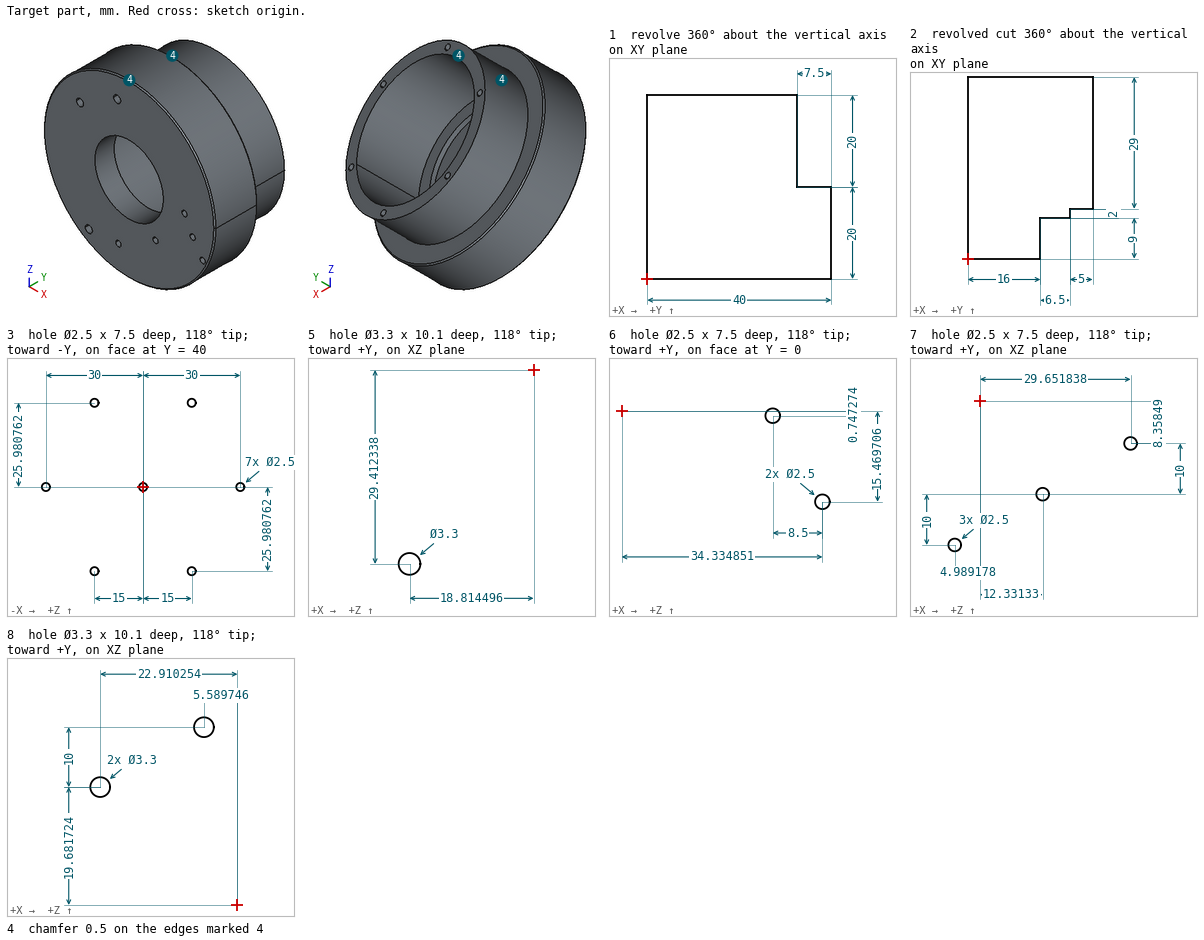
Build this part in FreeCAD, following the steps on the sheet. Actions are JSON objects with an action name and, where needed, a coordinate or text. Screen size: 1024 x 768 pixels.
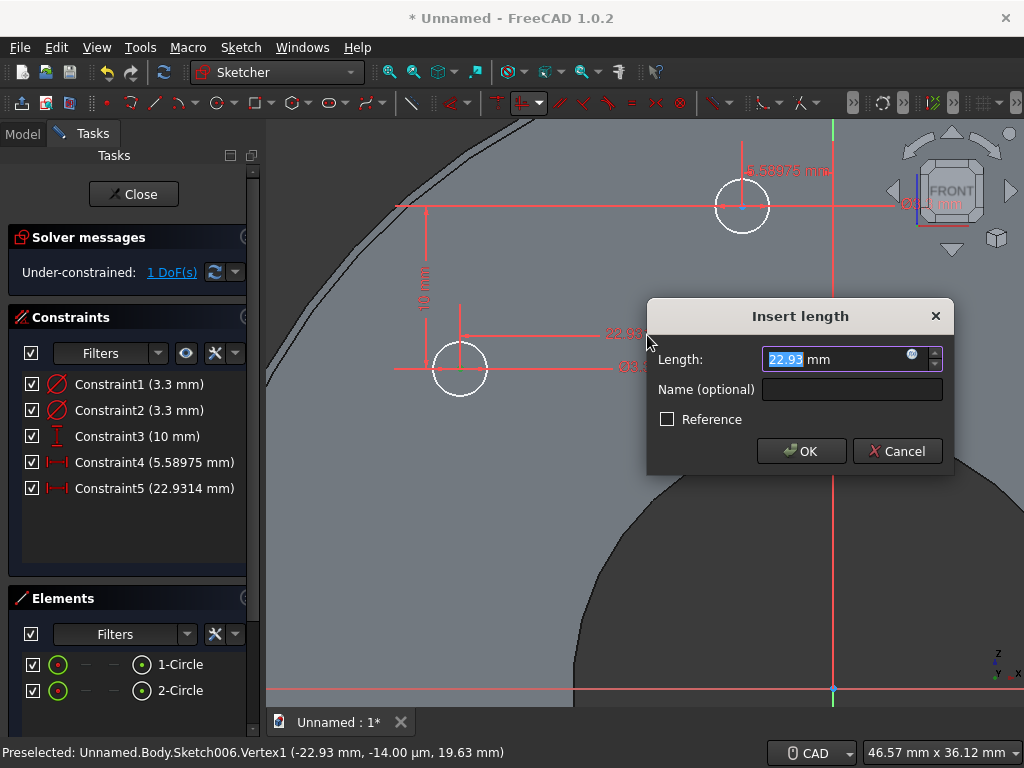
{"action": "type", "text": "22.910254"}
{"action": "key", "text": "Return"}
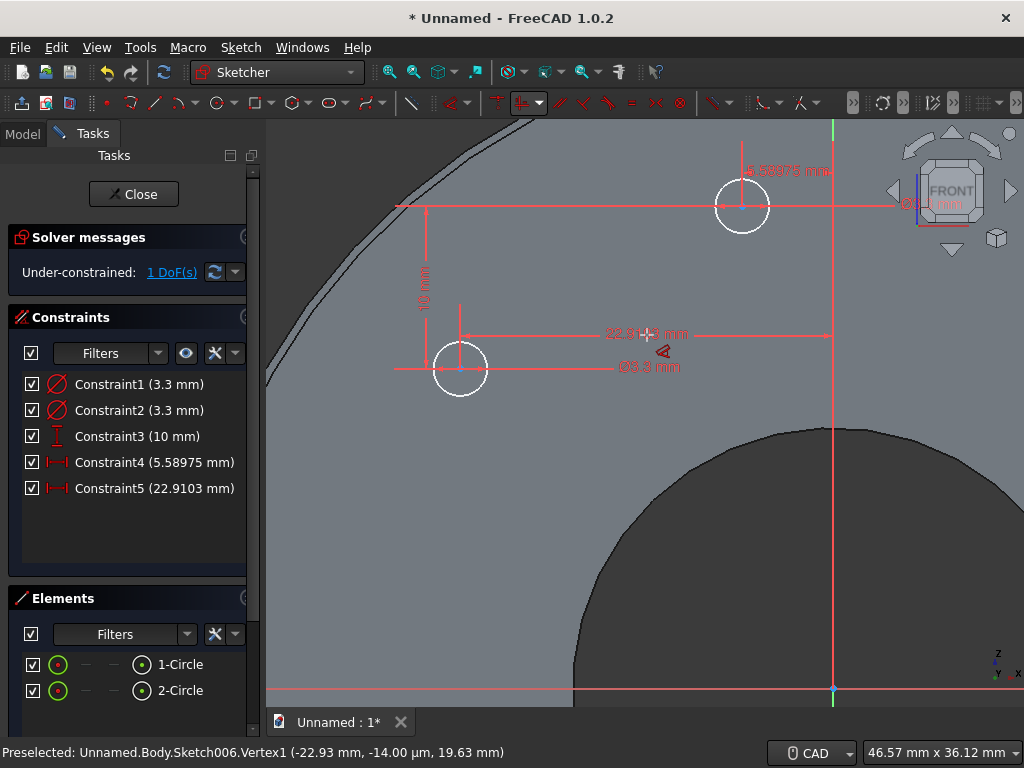
{"action": "left_click", "coordinate": [460, 369]}
{"action": "left_click", "coordinate": [426, 524]}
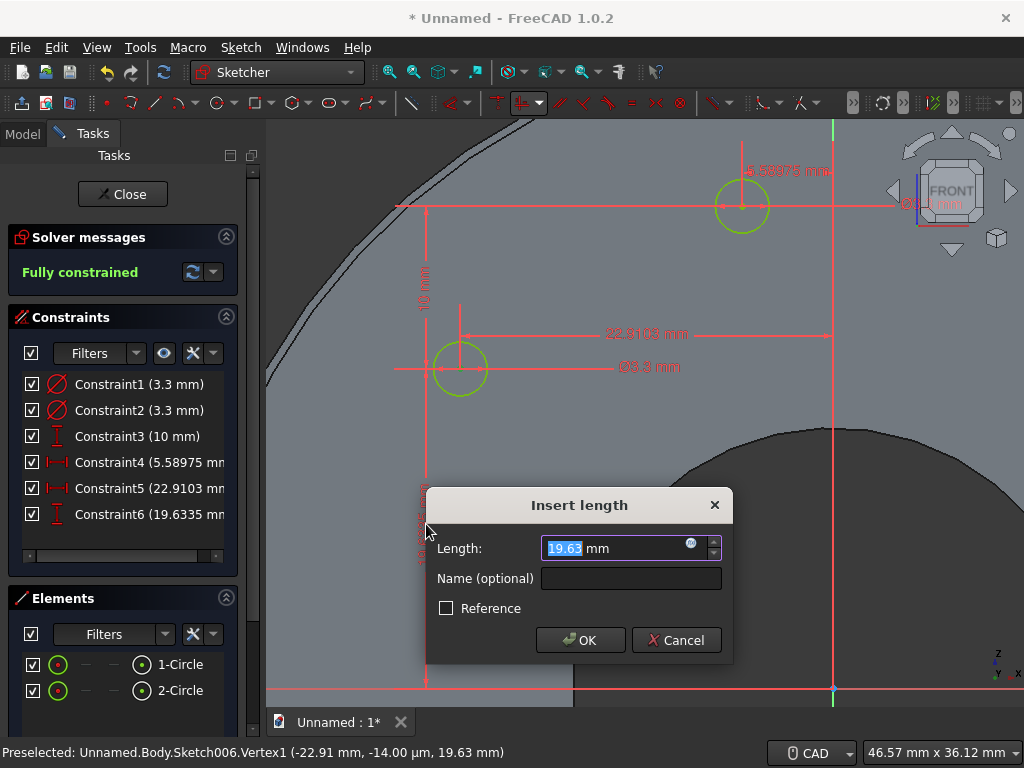
{"action": "type", "text": "19.681724"}
{"action": "key", "text": "Return"}
{"action": "key", "text": "Escape"}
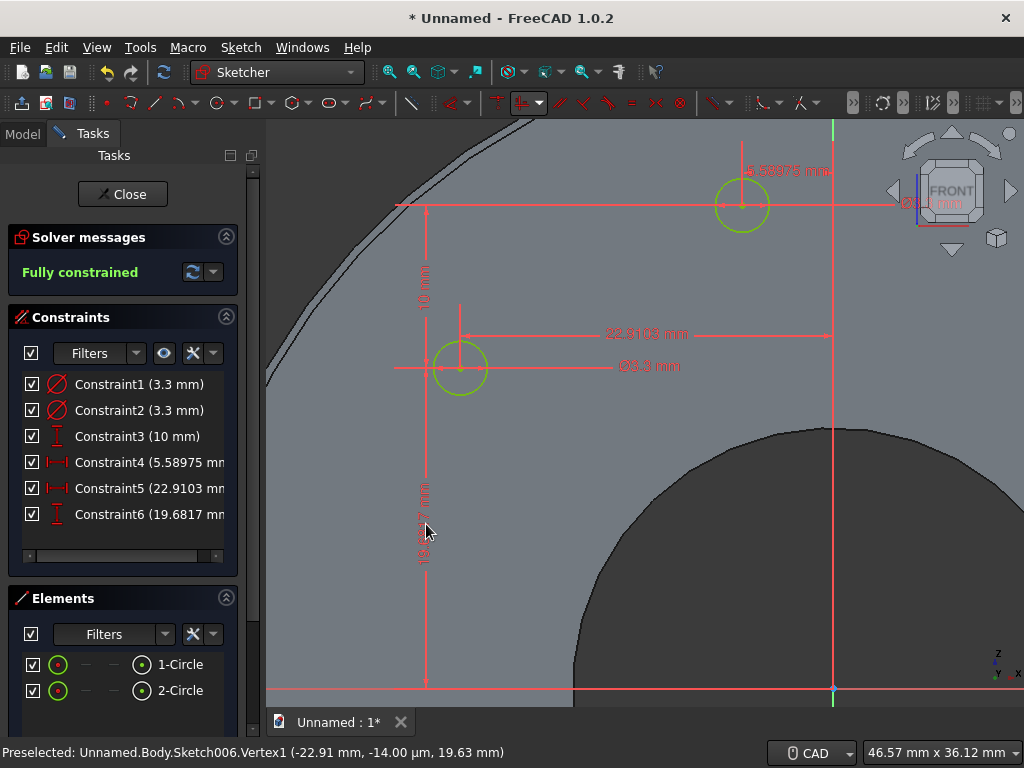
{"action": "left_click", "coordinate": [123, 194]}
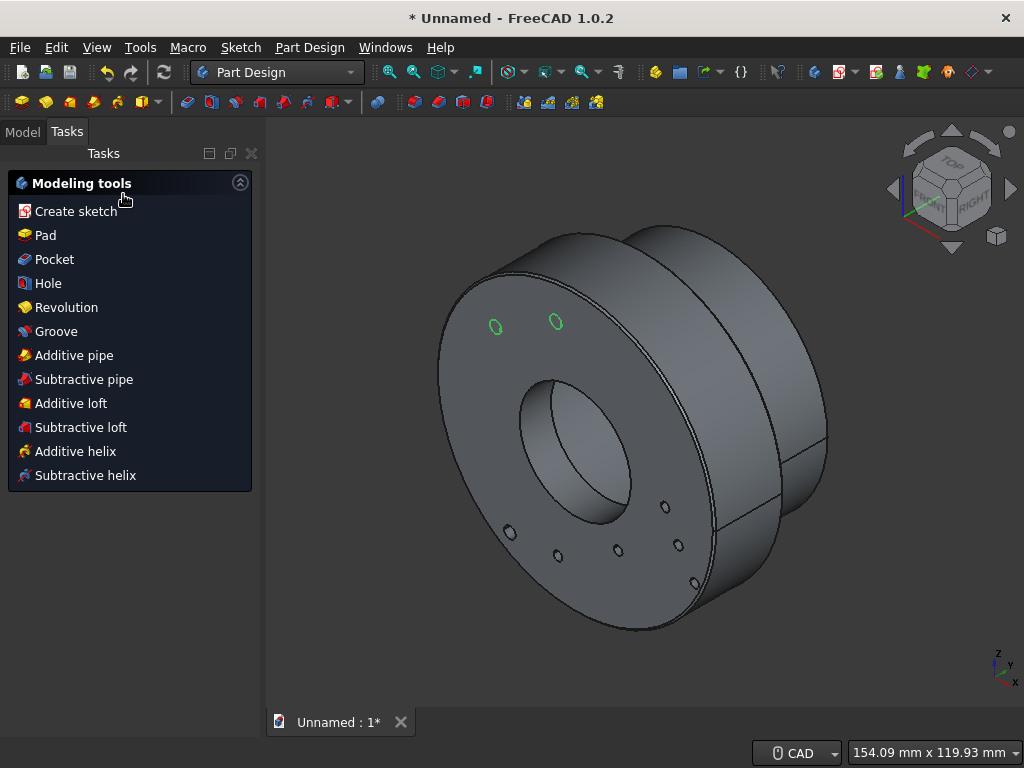
{"action": "left_click", "coordinate": [212, 102]}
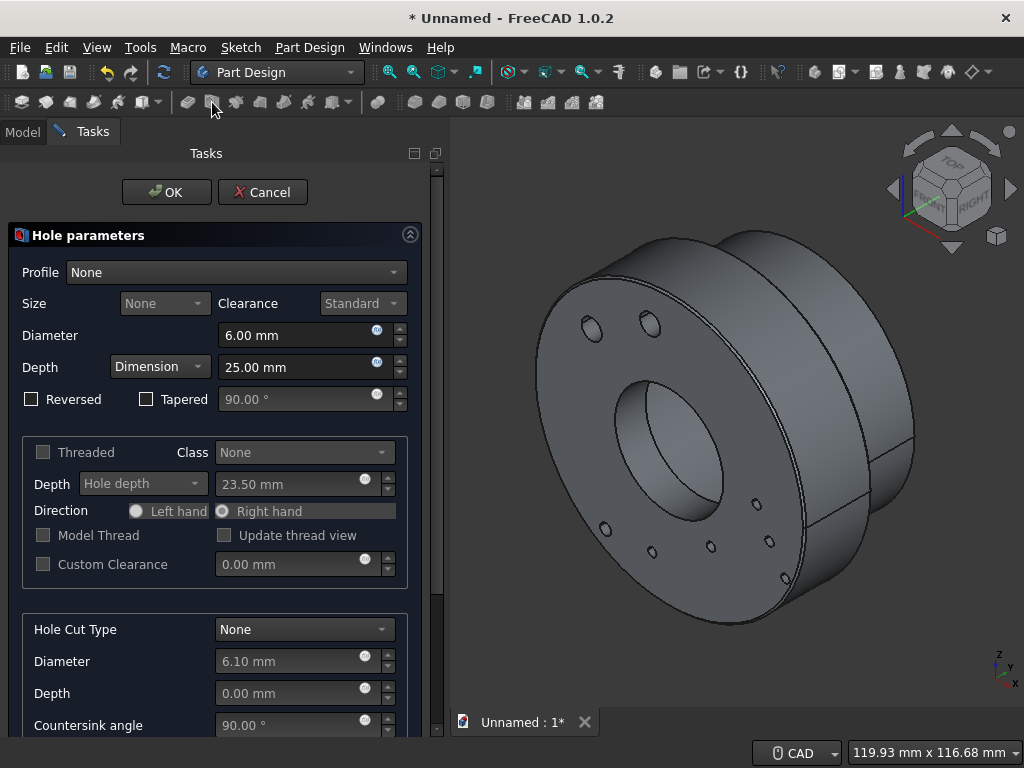
{"action": "triple_click", "coordinate": [305, 335]}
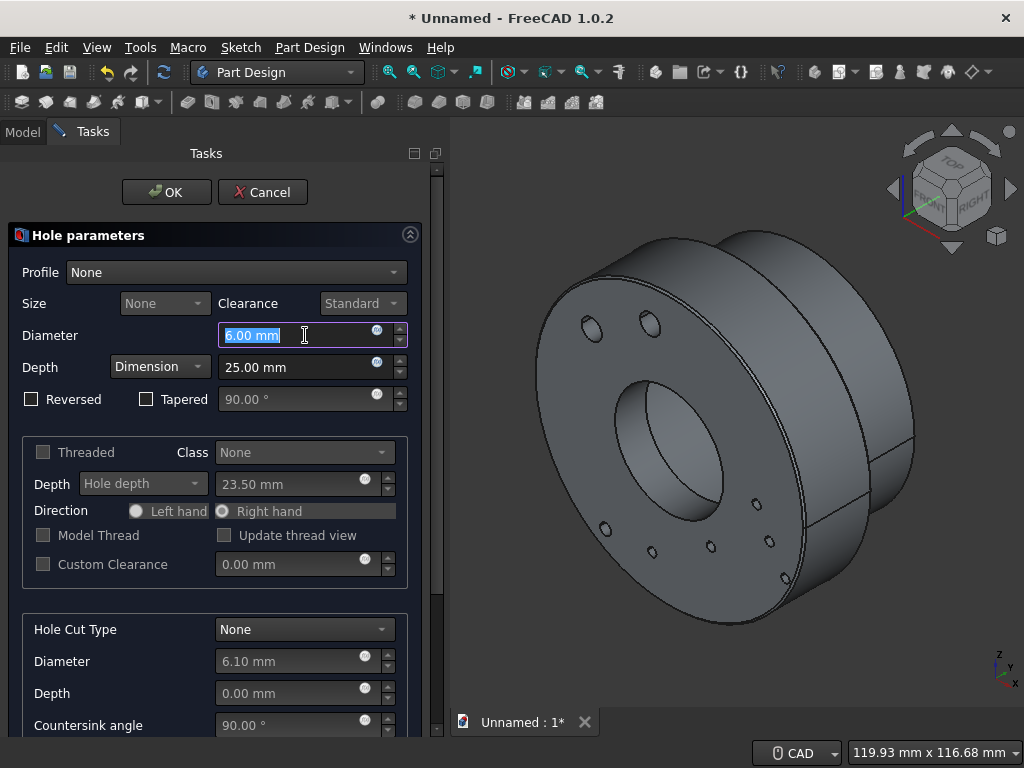
{"action": "type", "text": "3.3"}
{"action": "key", "text": "Tab"}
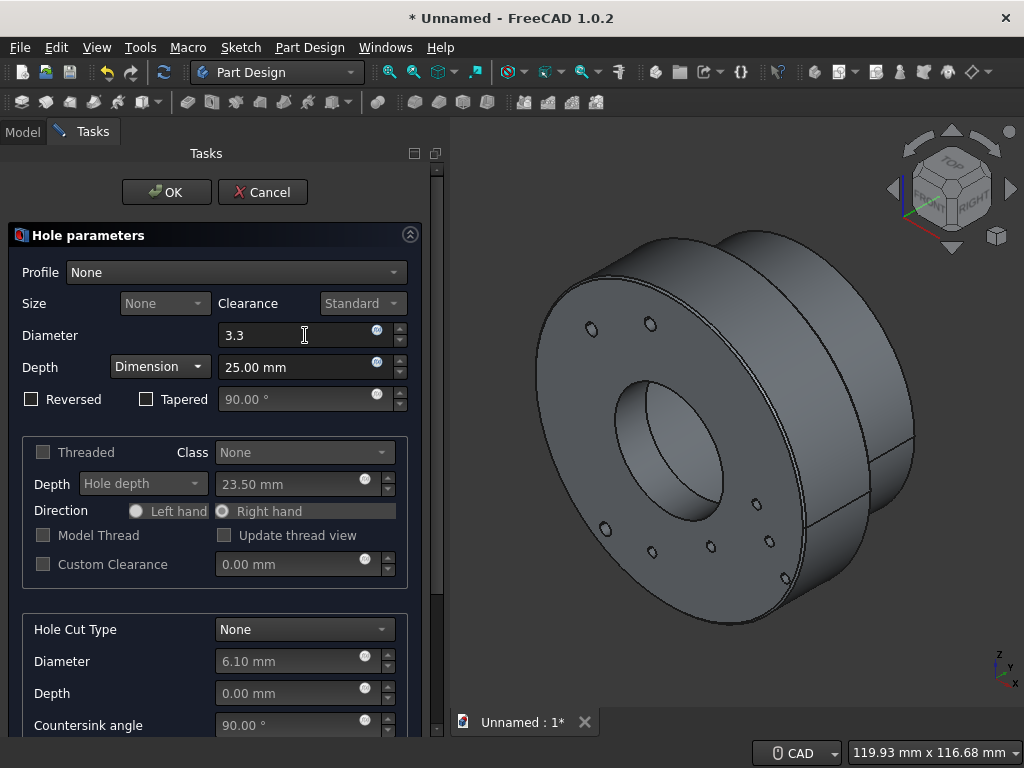
{"action": "triple_click", "coordinate": [305, 367]}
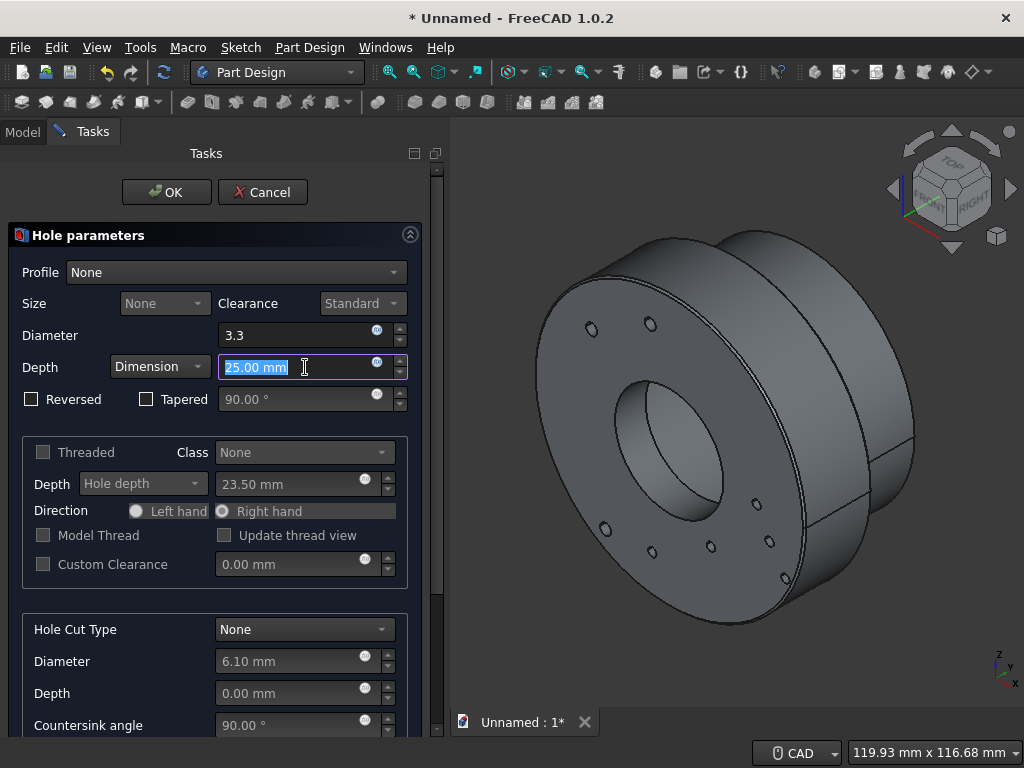
{"action": "type", "text": "10.1"}
{"action": "key", "text": "Tab"}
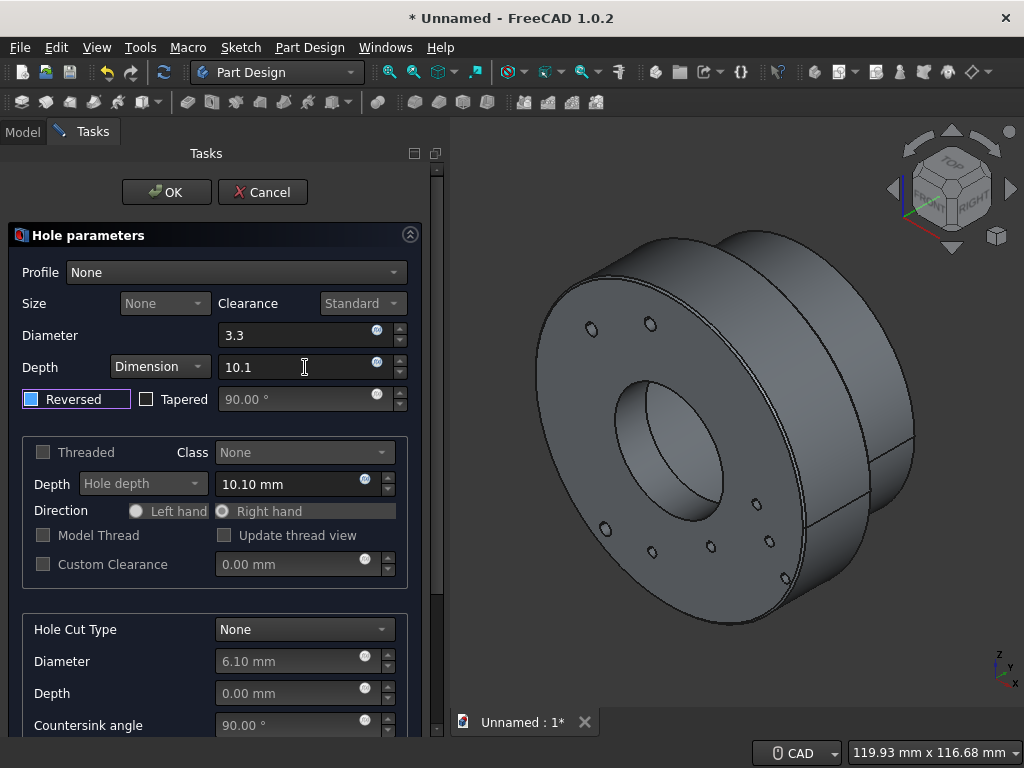
{"action": "left_click", "coordinate": [167, 192]}